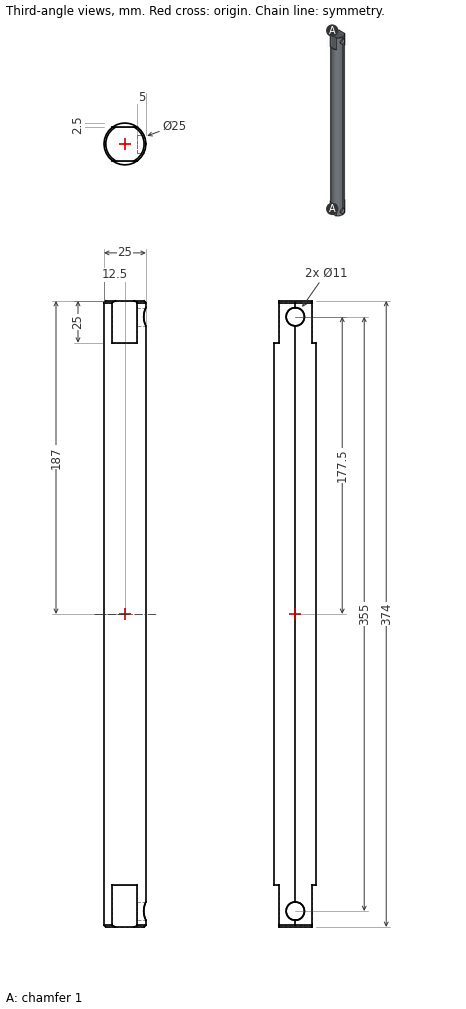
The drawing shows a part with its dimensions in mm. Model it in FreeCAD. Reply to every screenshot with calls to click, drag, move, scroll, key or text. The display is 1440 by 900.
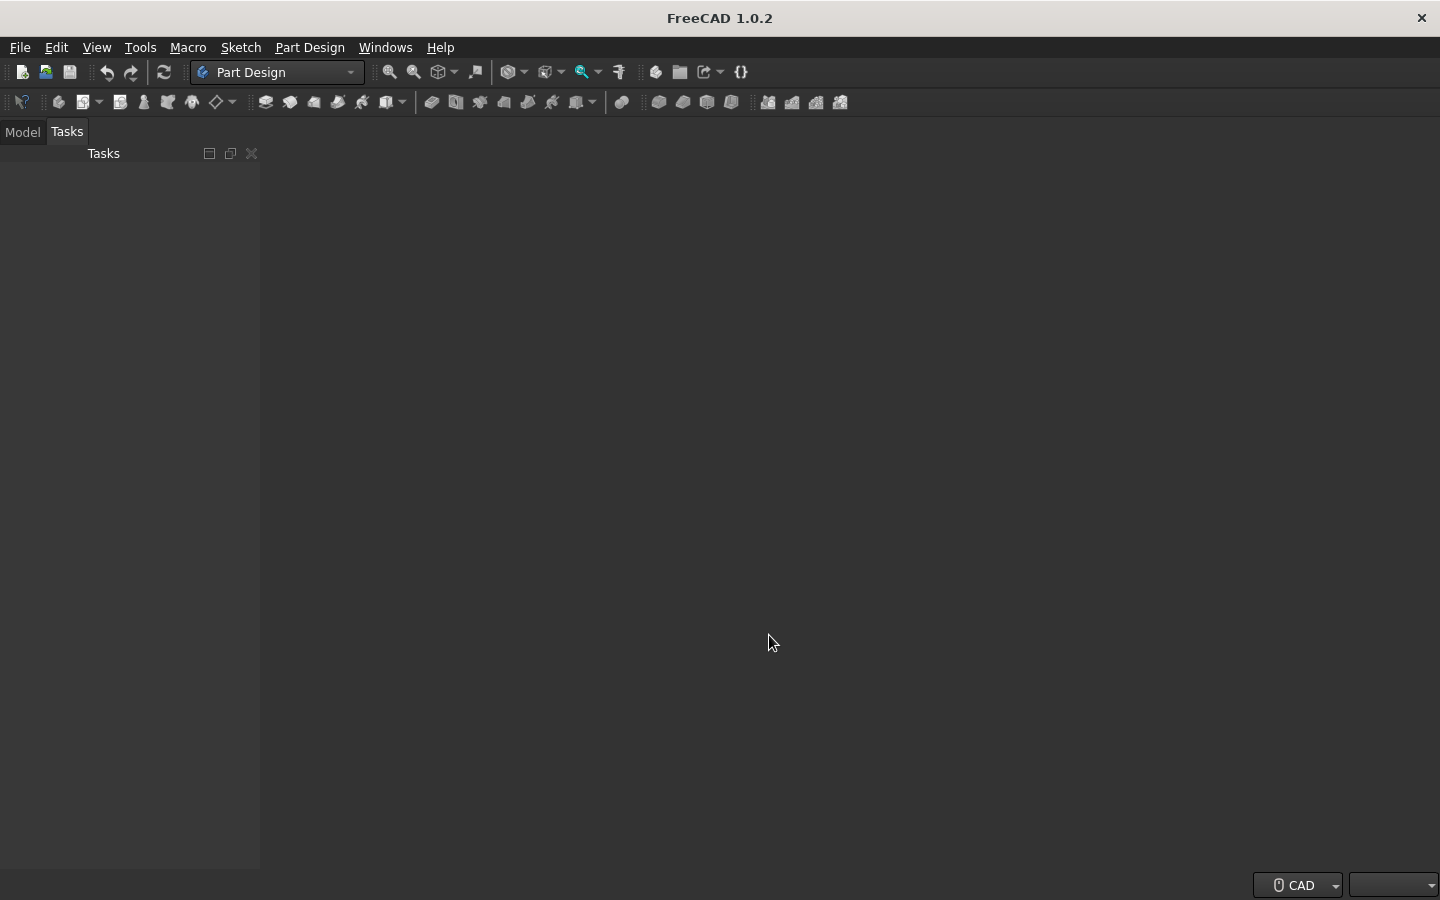
click(22, 72)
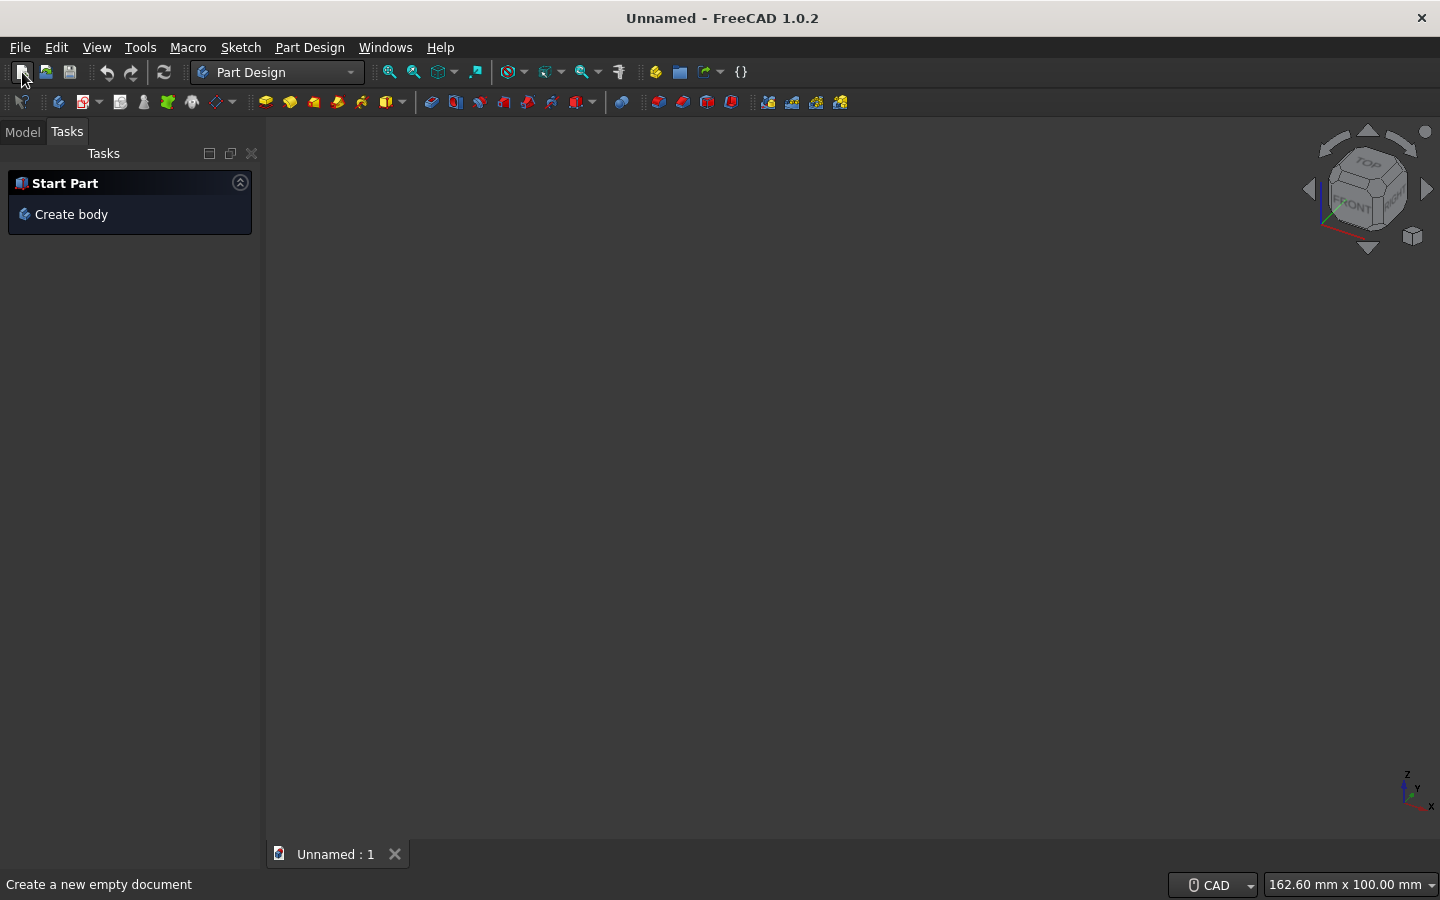
click(84, 102)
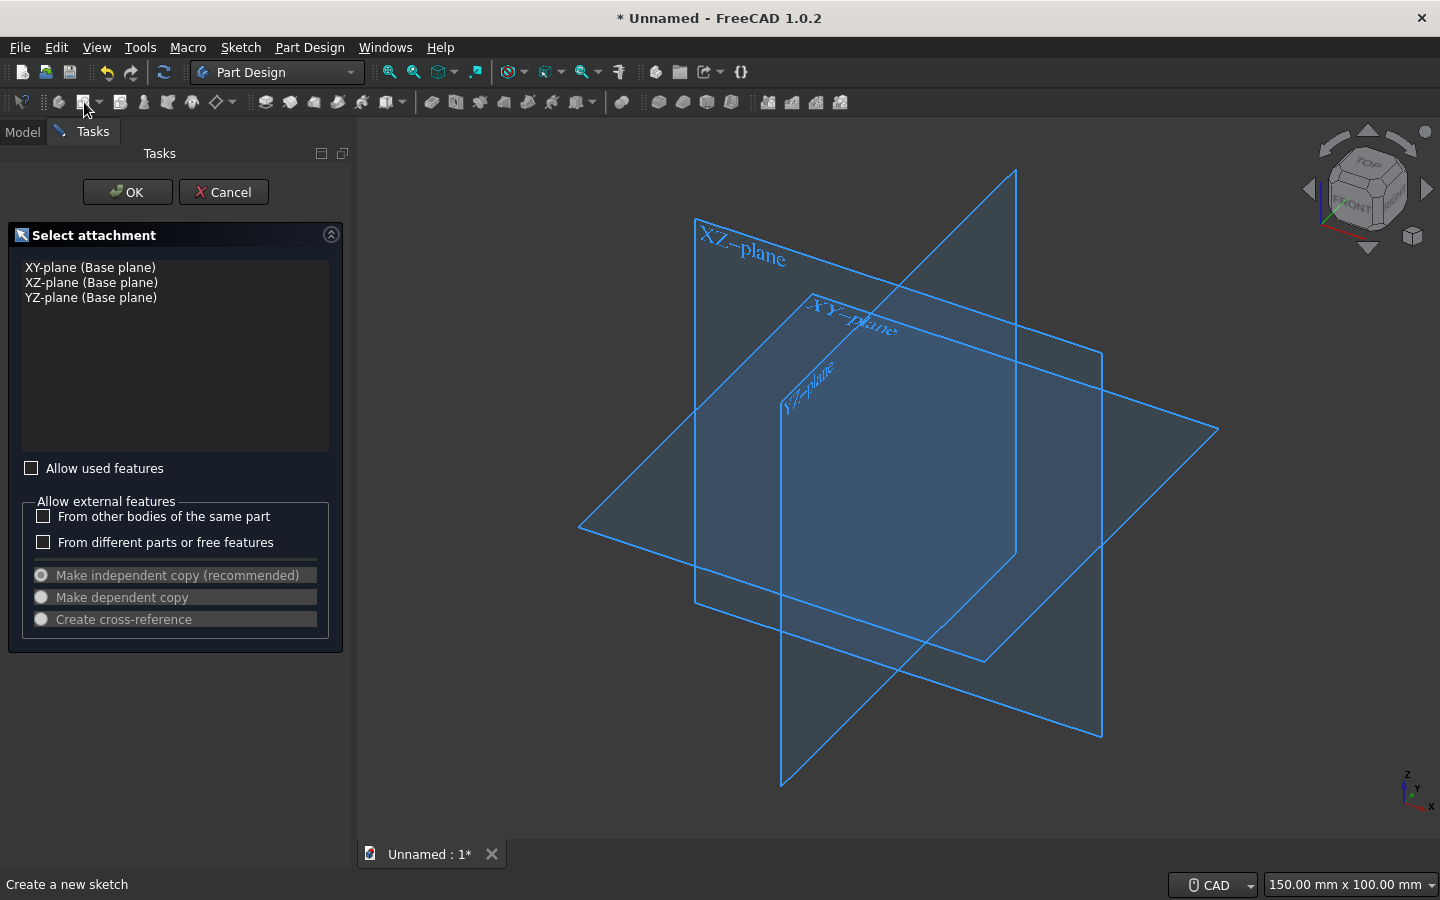
click(82, 268)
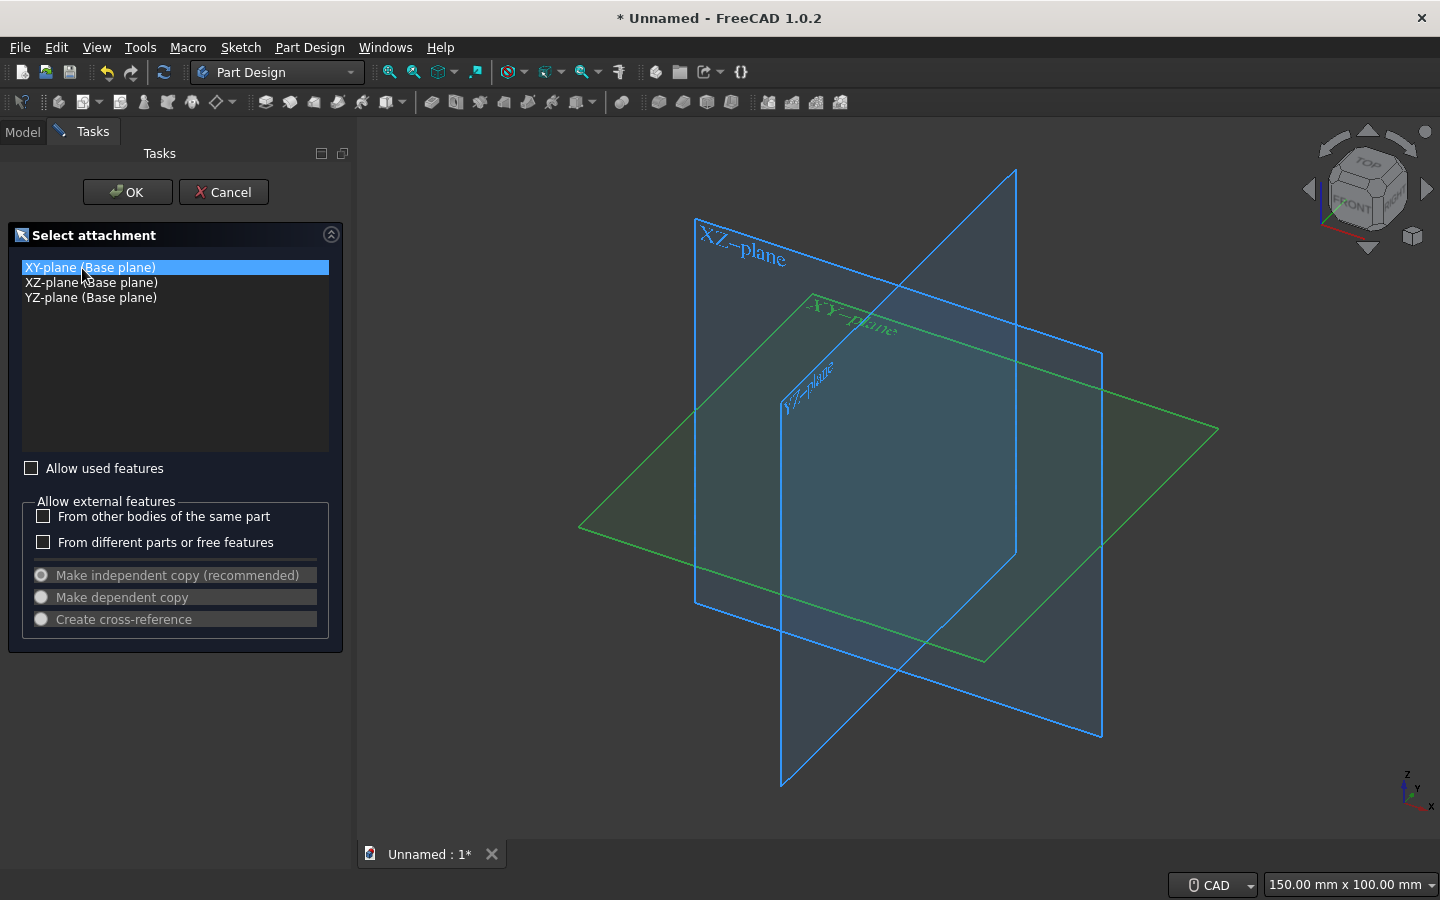
click(128, 192)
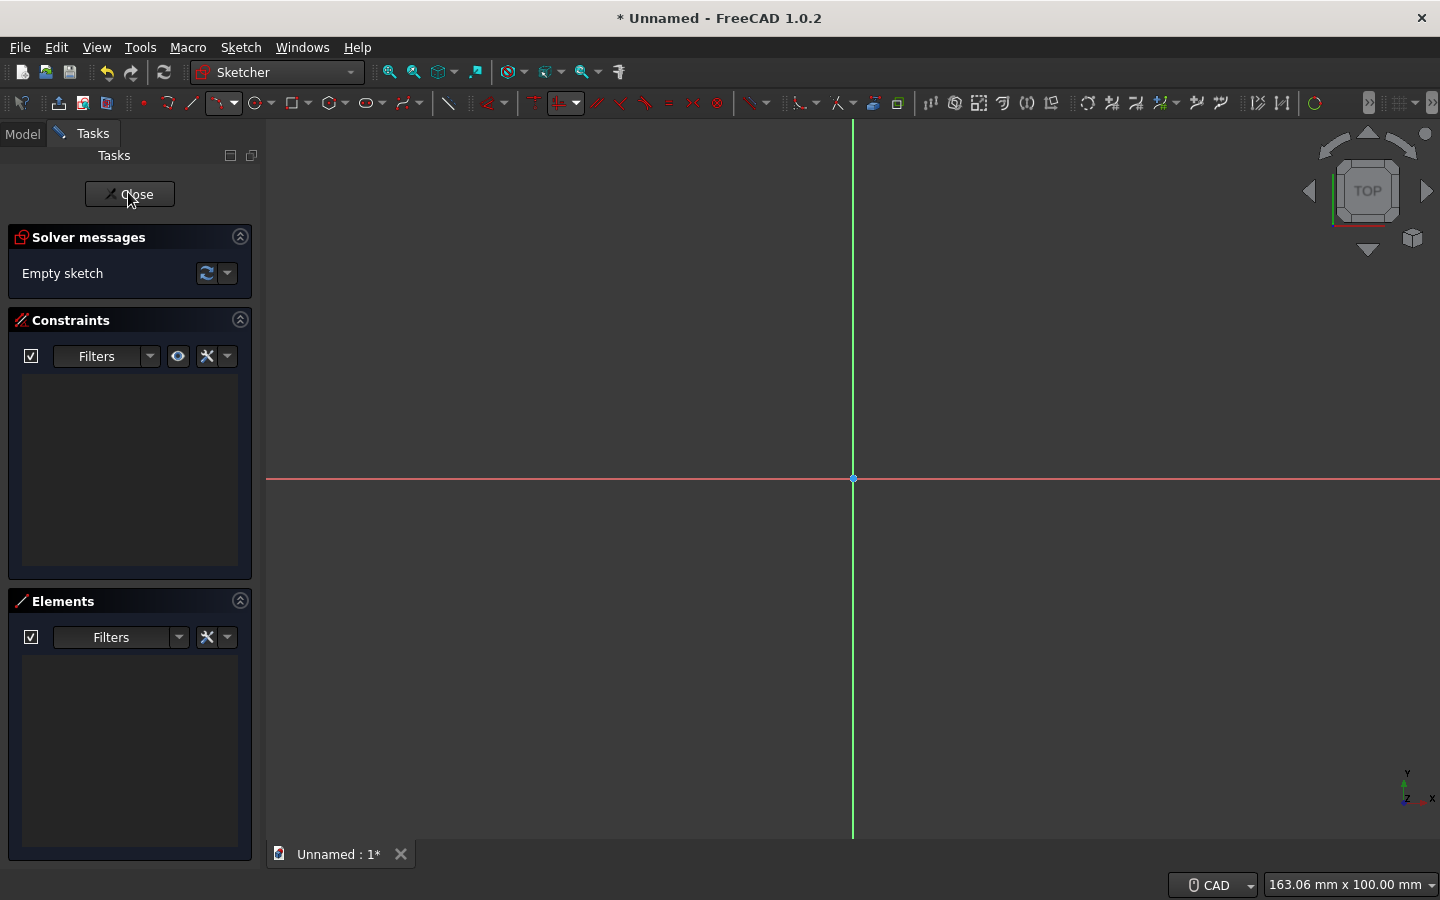
scroll(893, 479, up, 5)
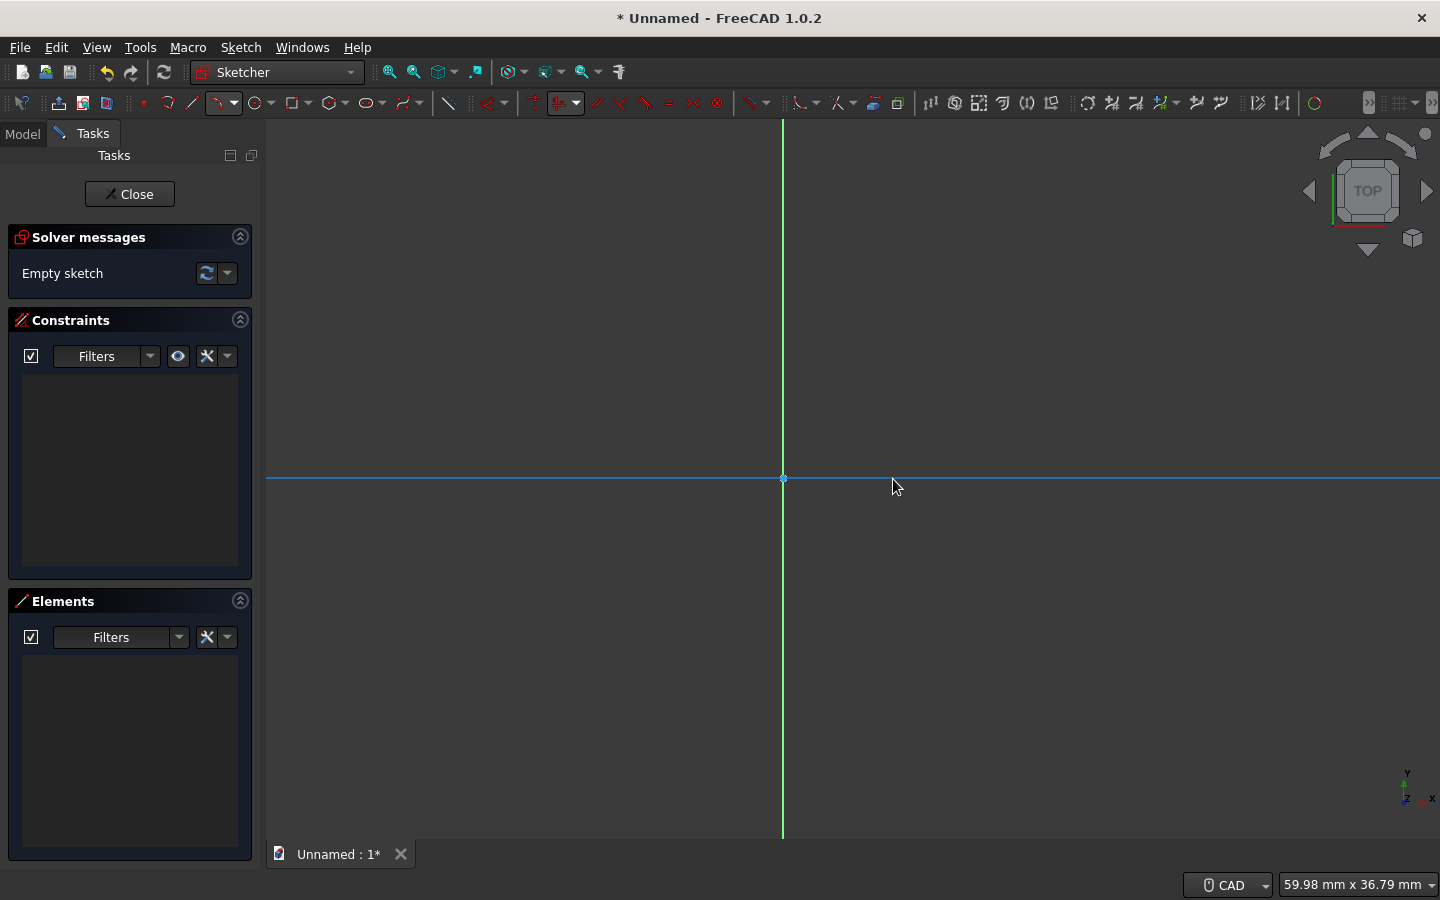
click(256, 104)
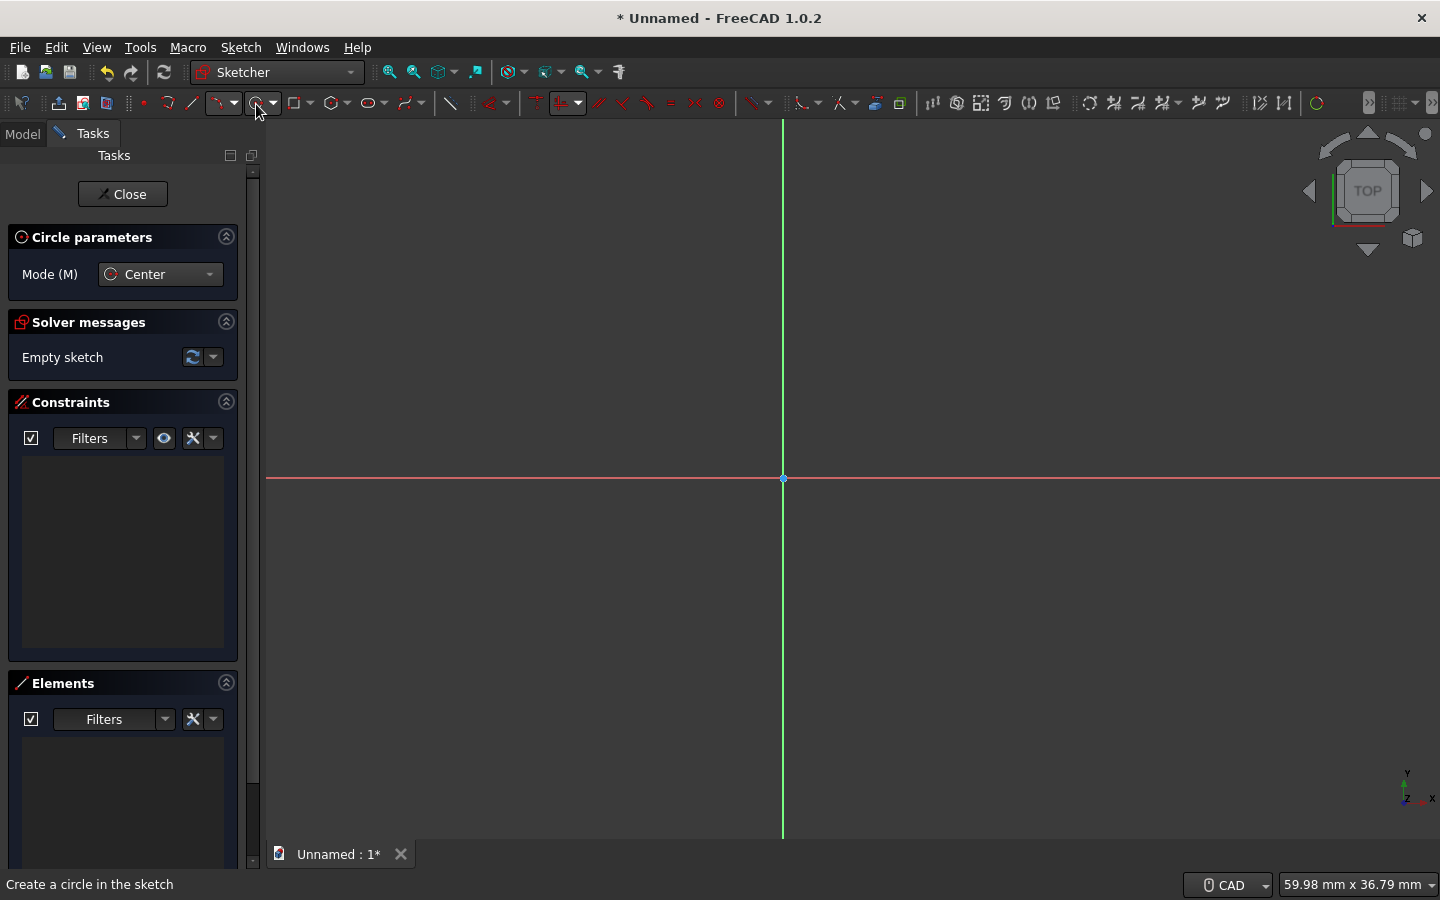
click(783, 478)
click(956, 305)
key(Escape)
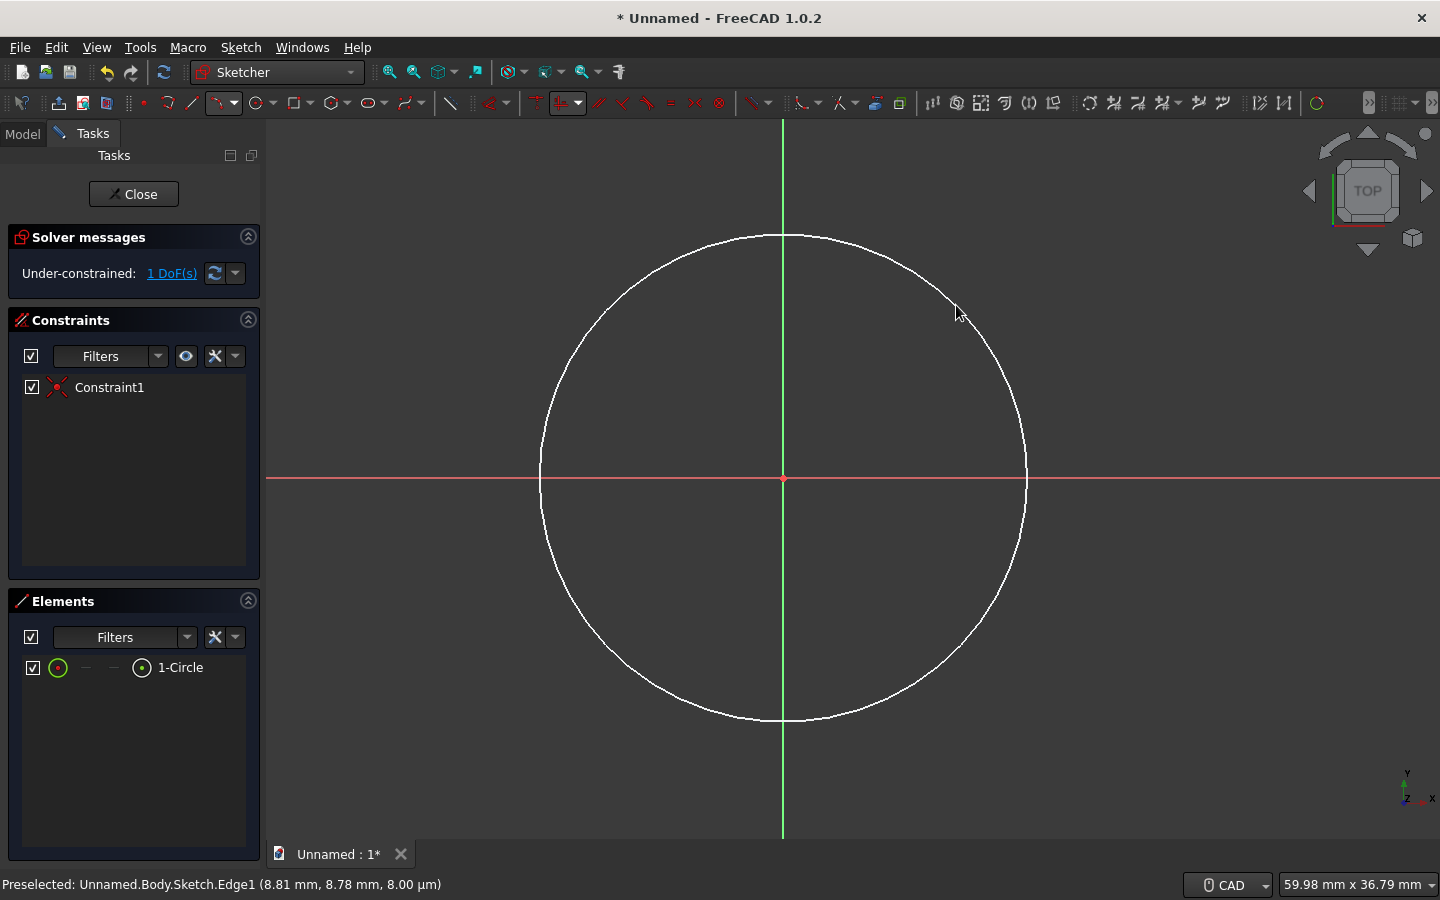
click(490, 104)